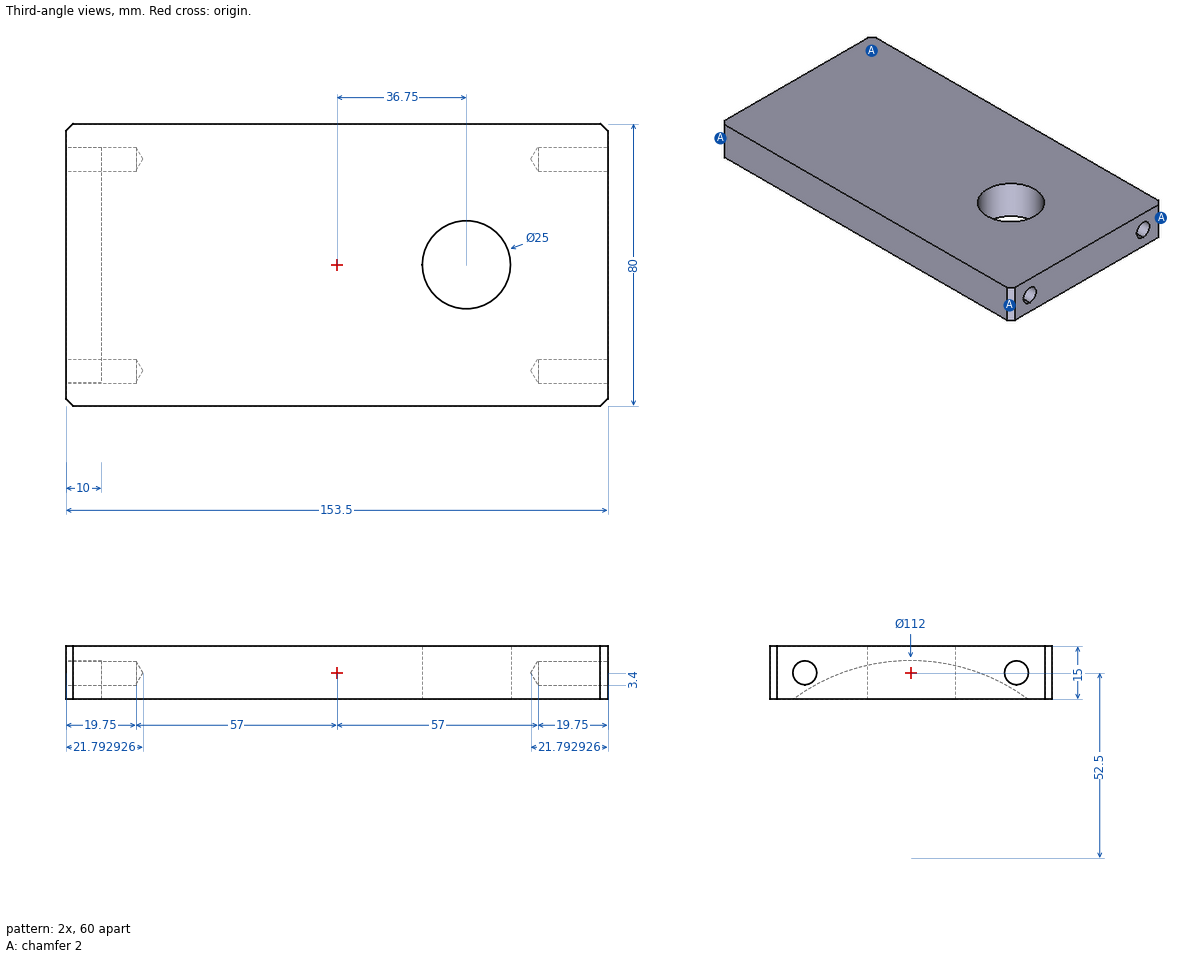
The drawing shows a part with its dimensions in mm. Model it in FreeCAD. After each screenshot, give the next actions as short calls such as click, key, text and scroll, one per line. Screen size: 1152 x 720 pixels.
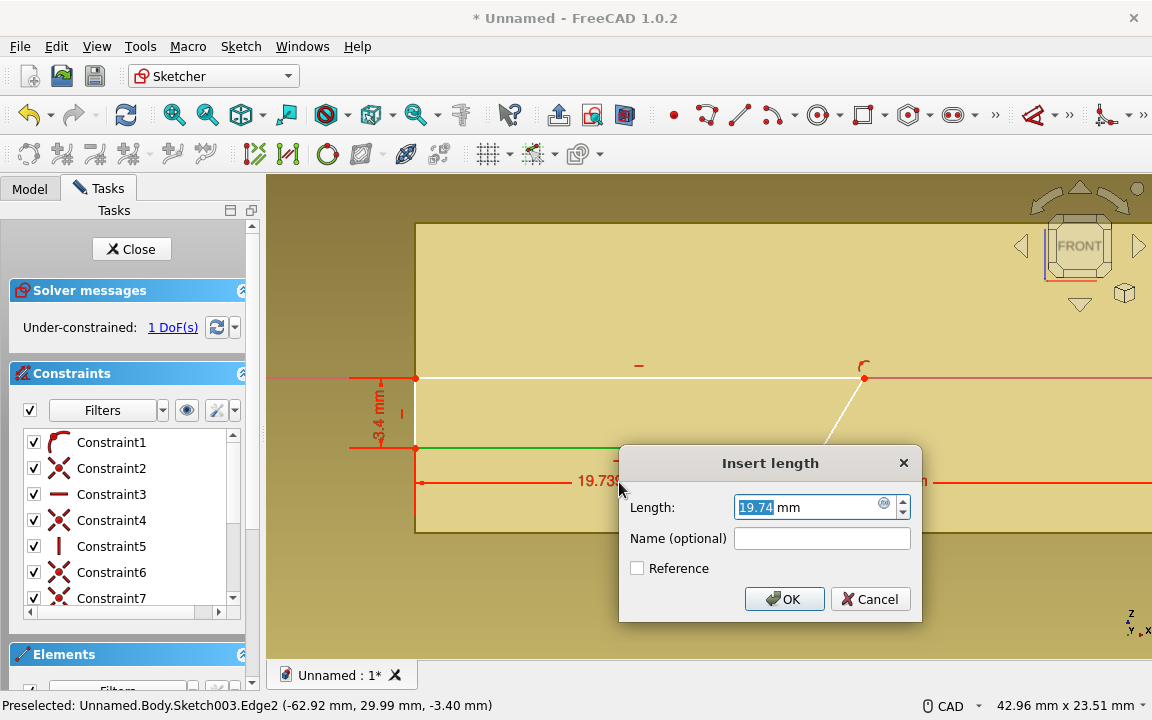
text(19.75)
key(Return)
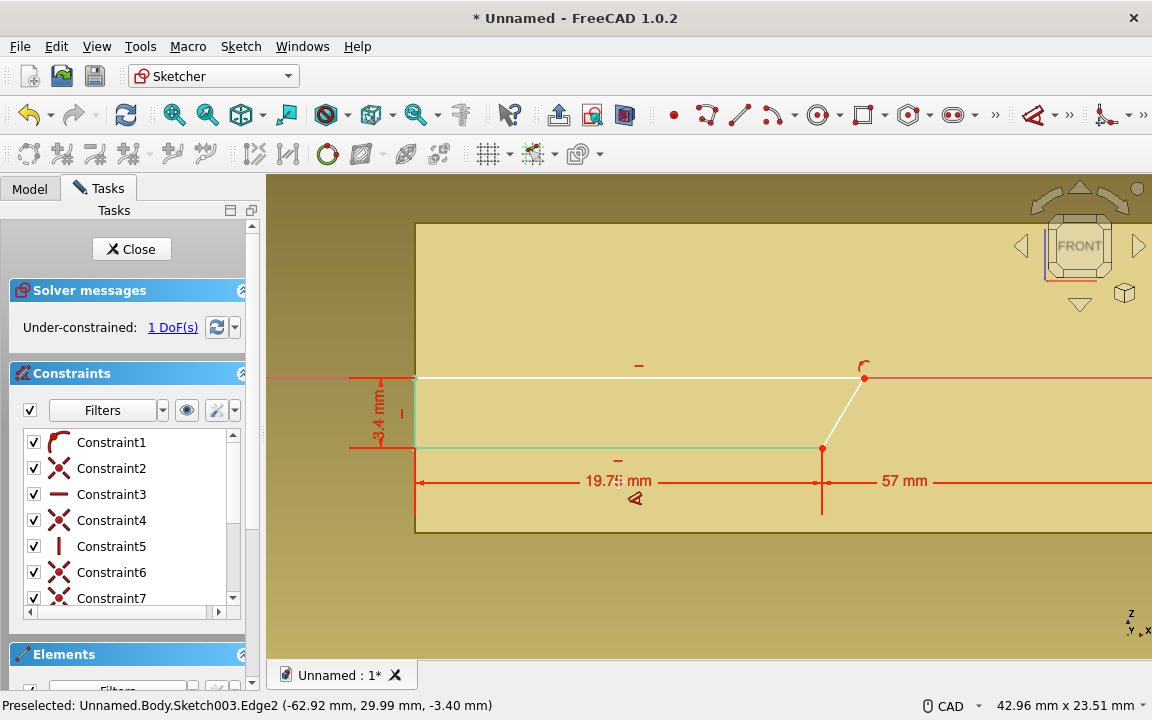
click(550, 378)
click(639, 344)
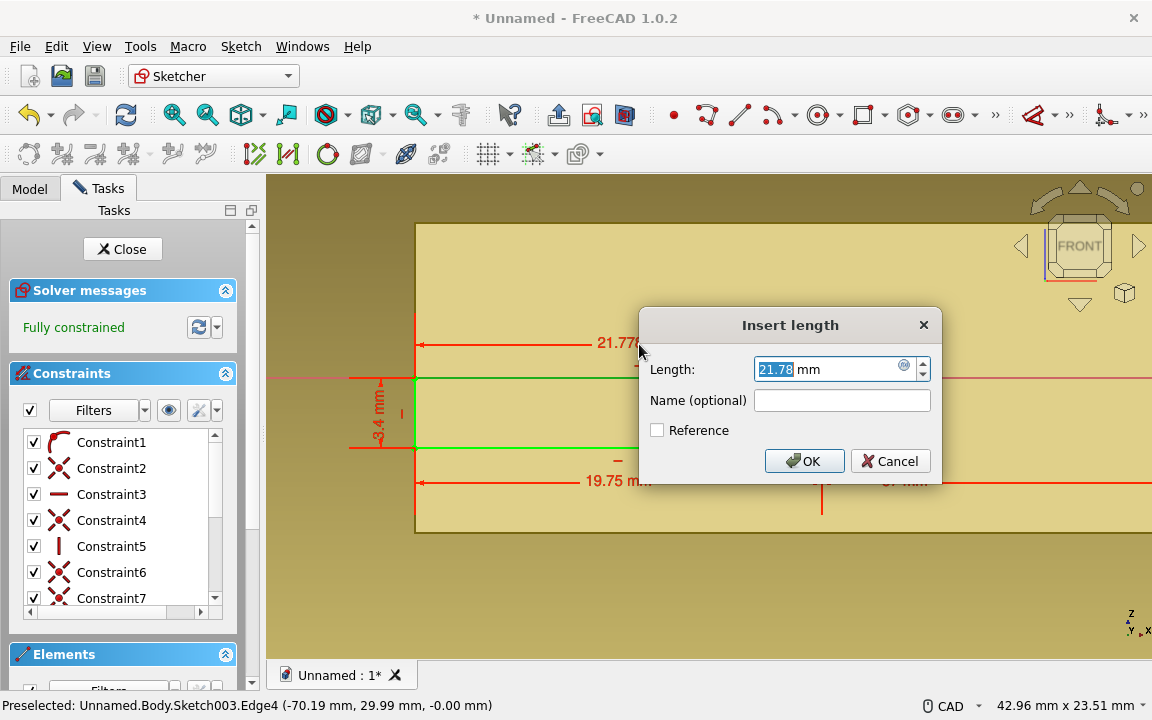
text(21.792926)
key(Return)
key(Escape)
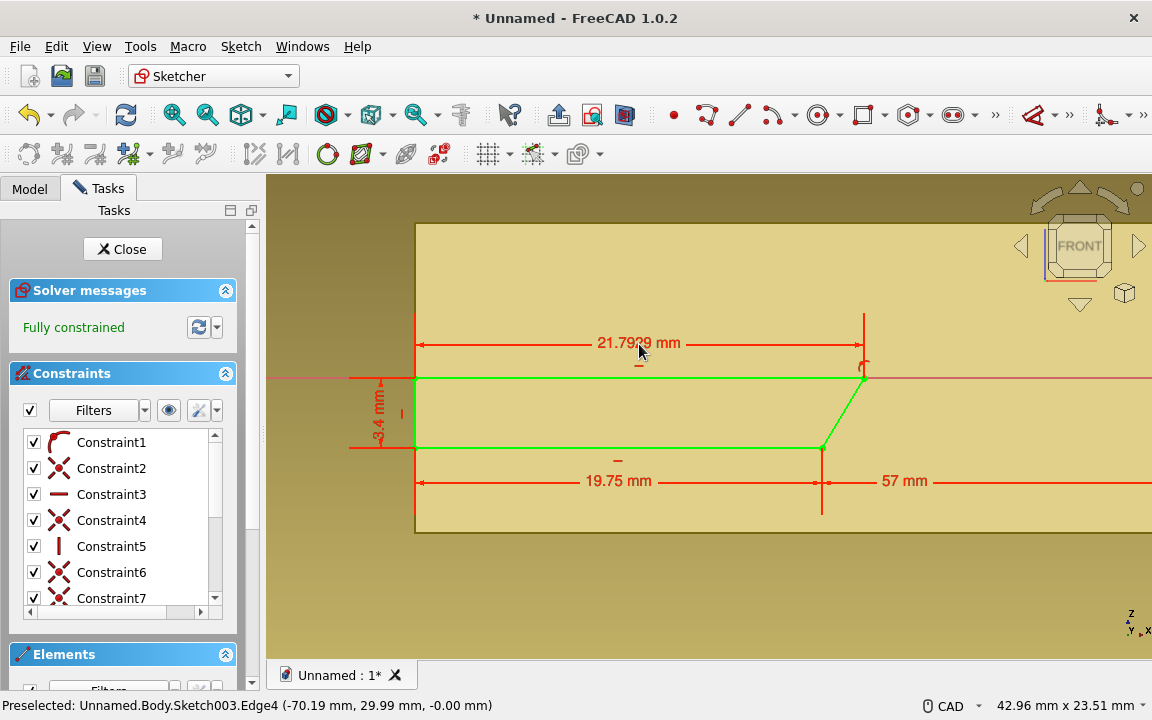
click(123, 249)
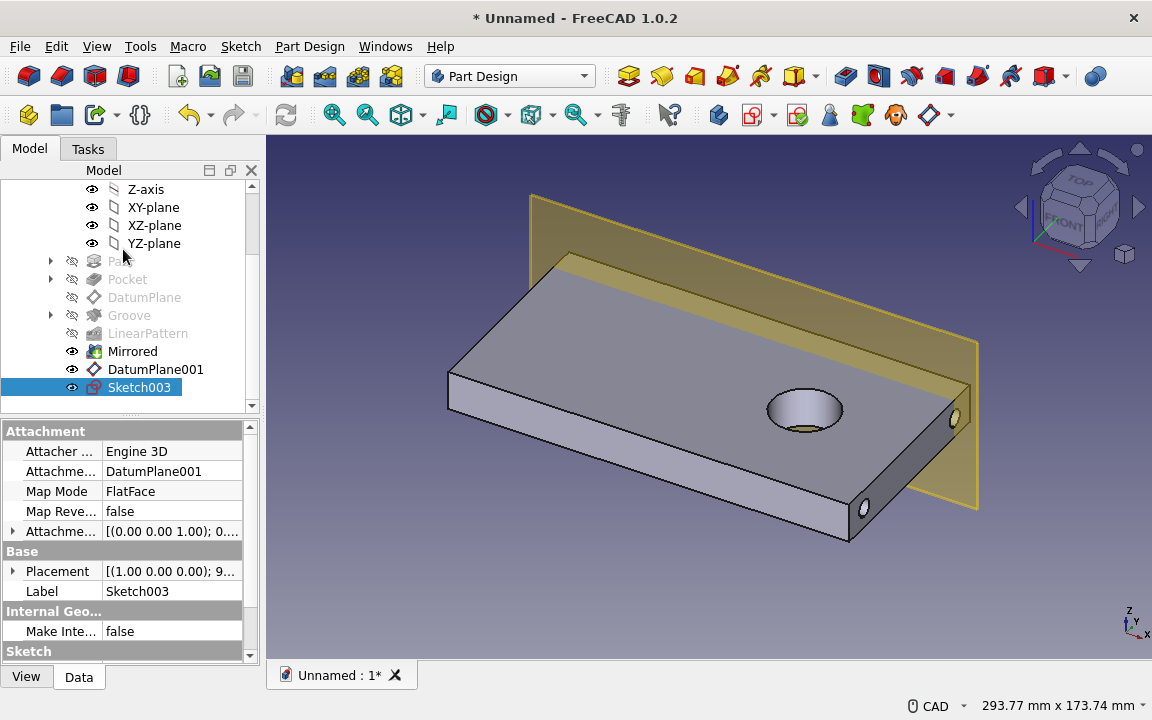
click(912, 76)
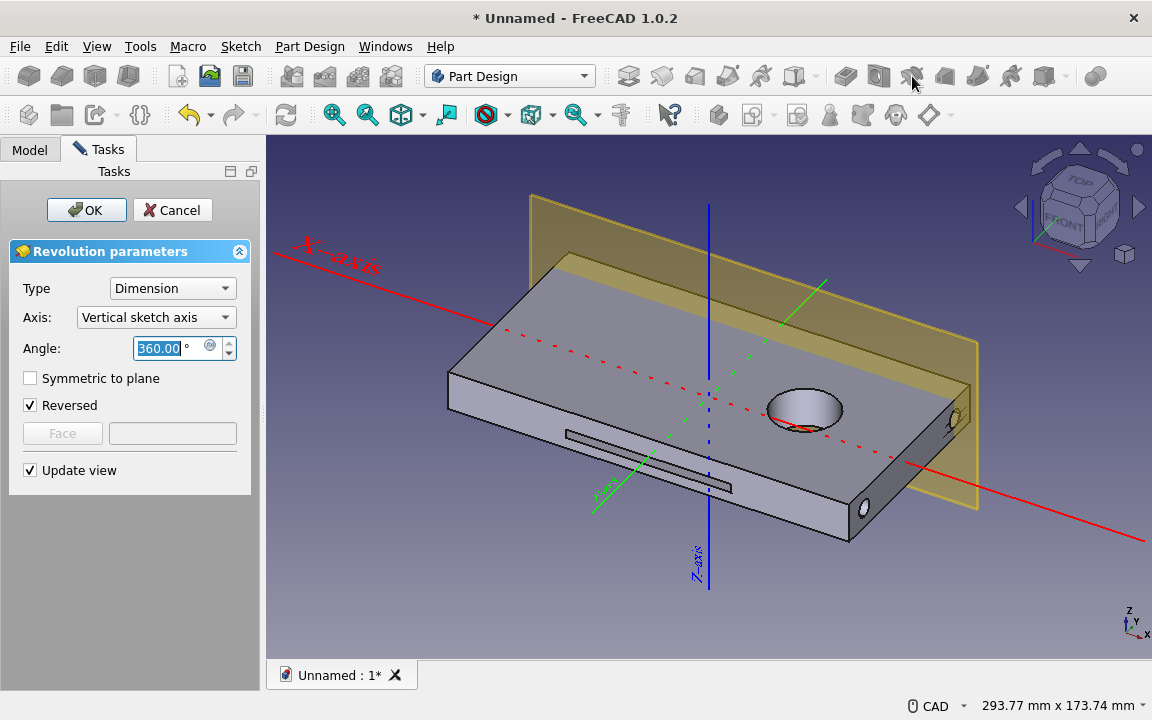
click(157, 318)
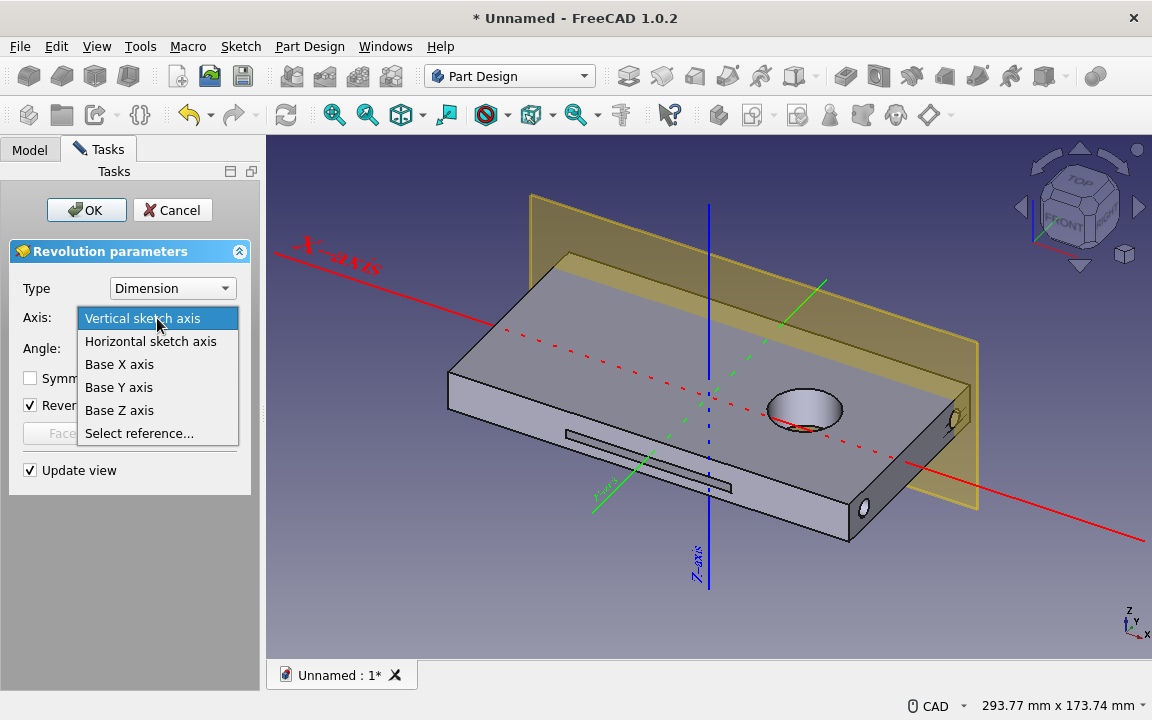
click(156, 342)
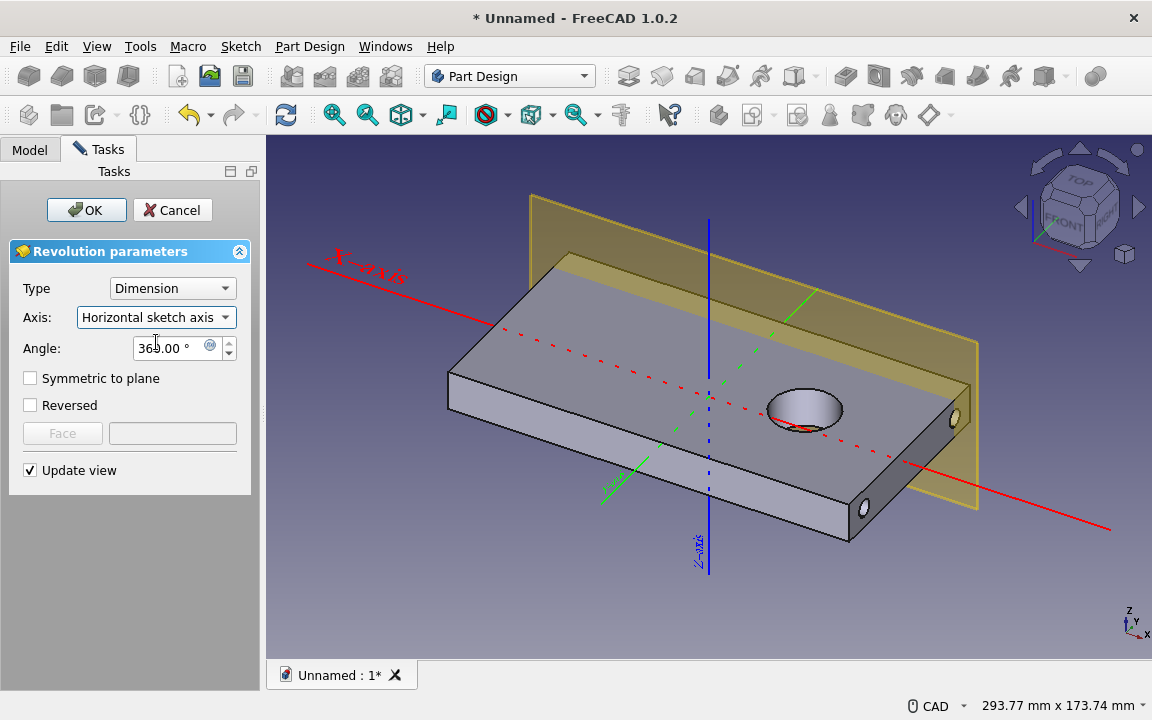
click(87, 210)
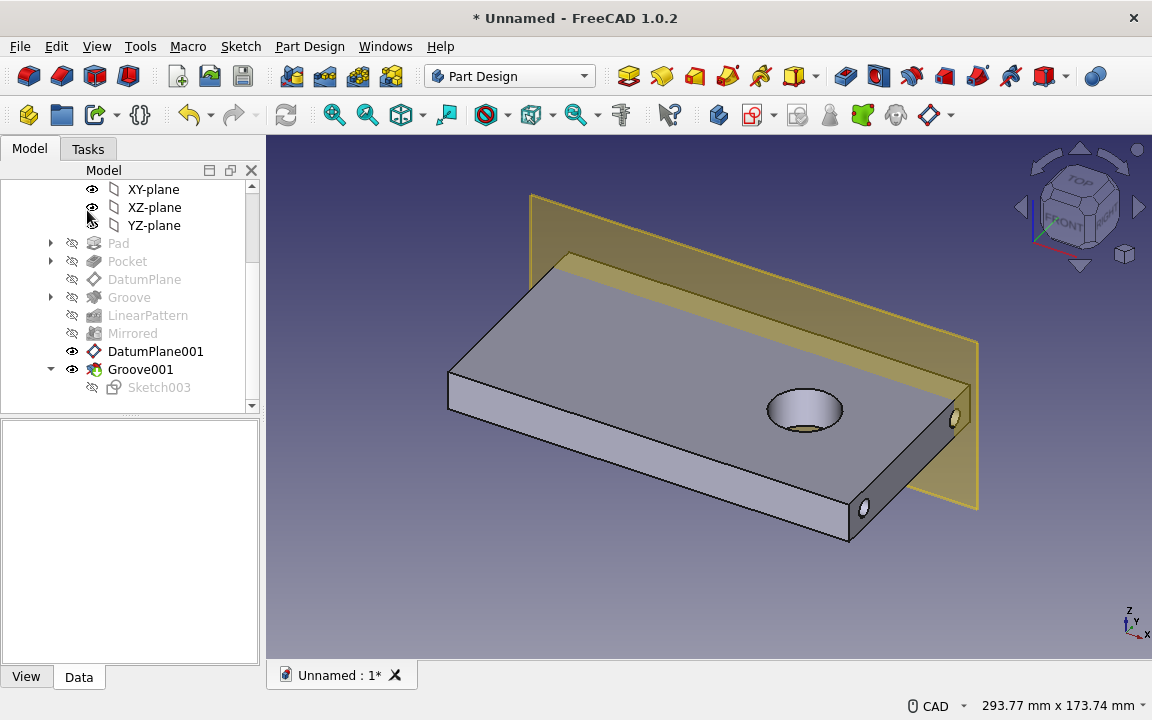
click(117, 351)
key(space)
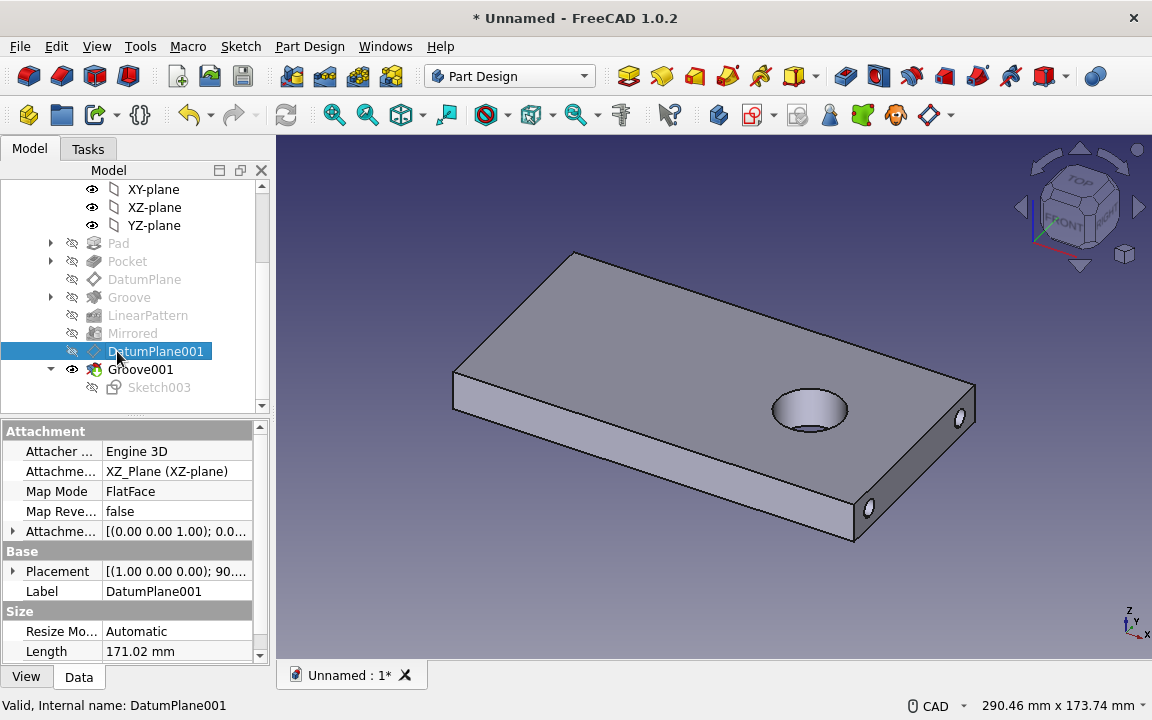
key(6)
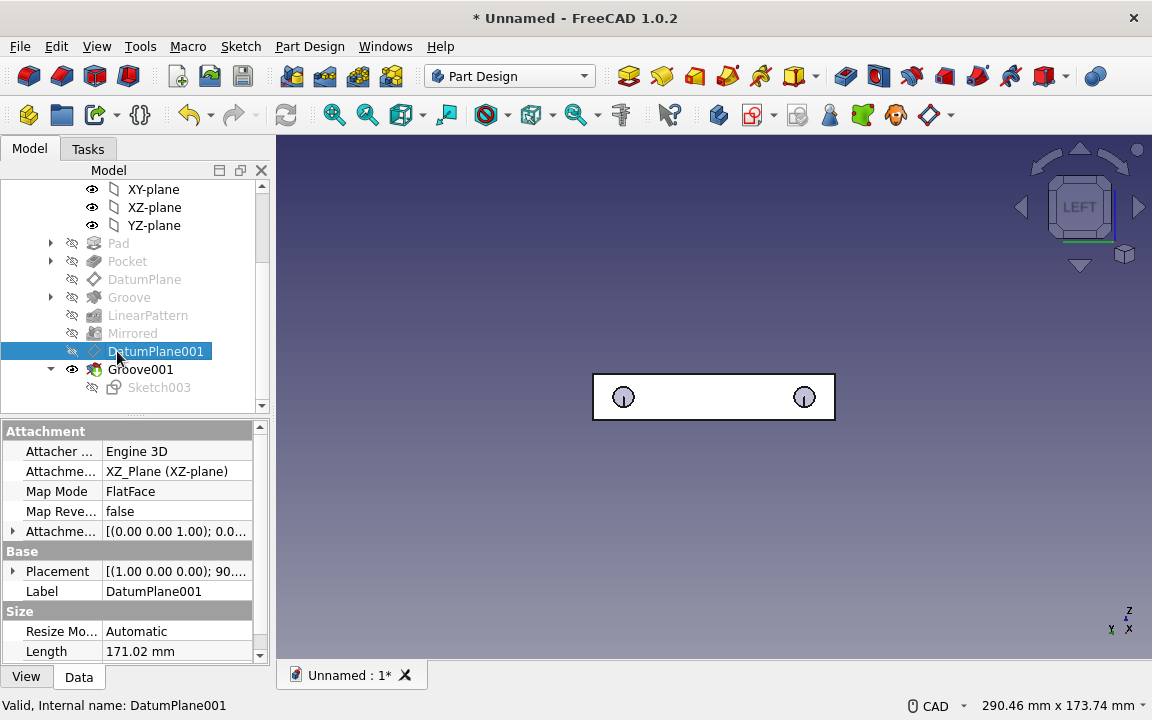
click(335, 116)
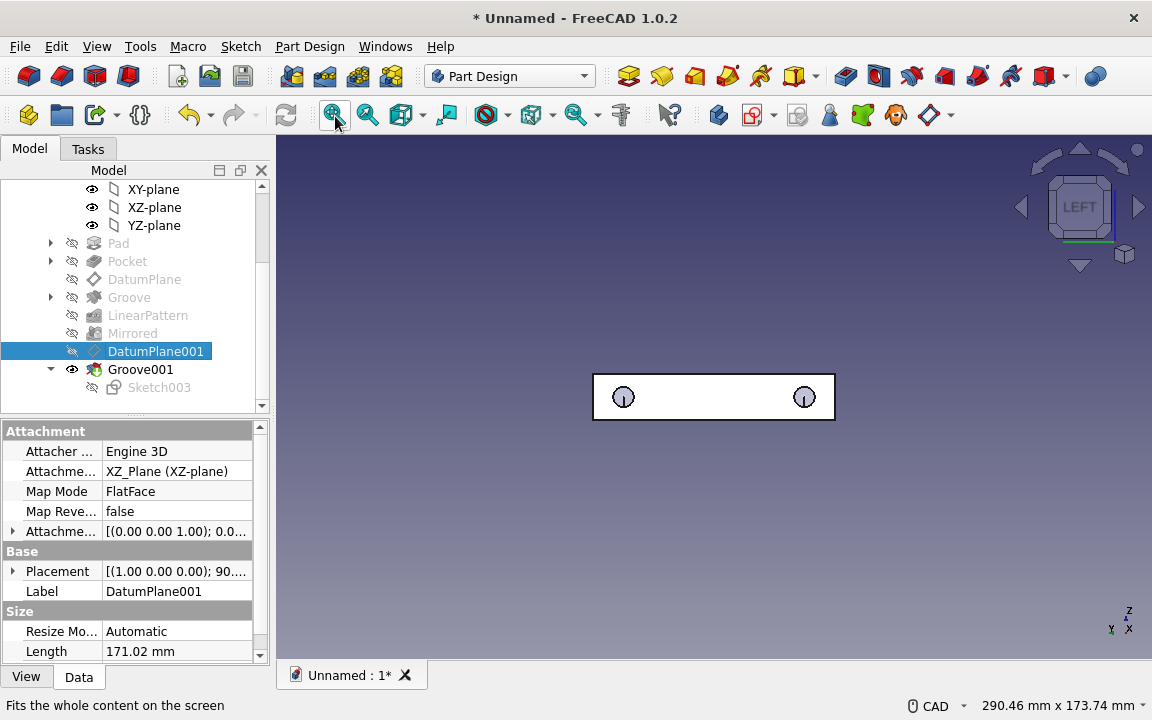
click(680, 396)